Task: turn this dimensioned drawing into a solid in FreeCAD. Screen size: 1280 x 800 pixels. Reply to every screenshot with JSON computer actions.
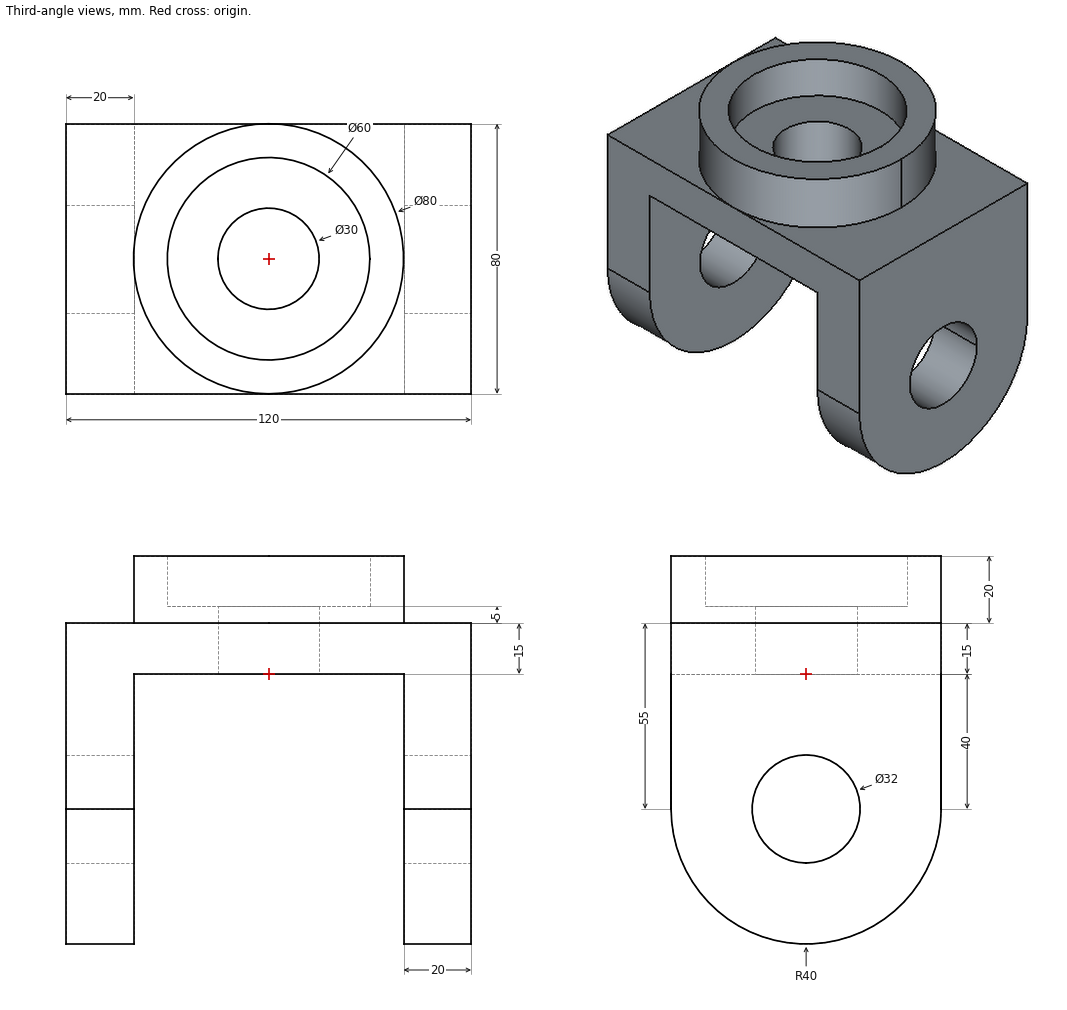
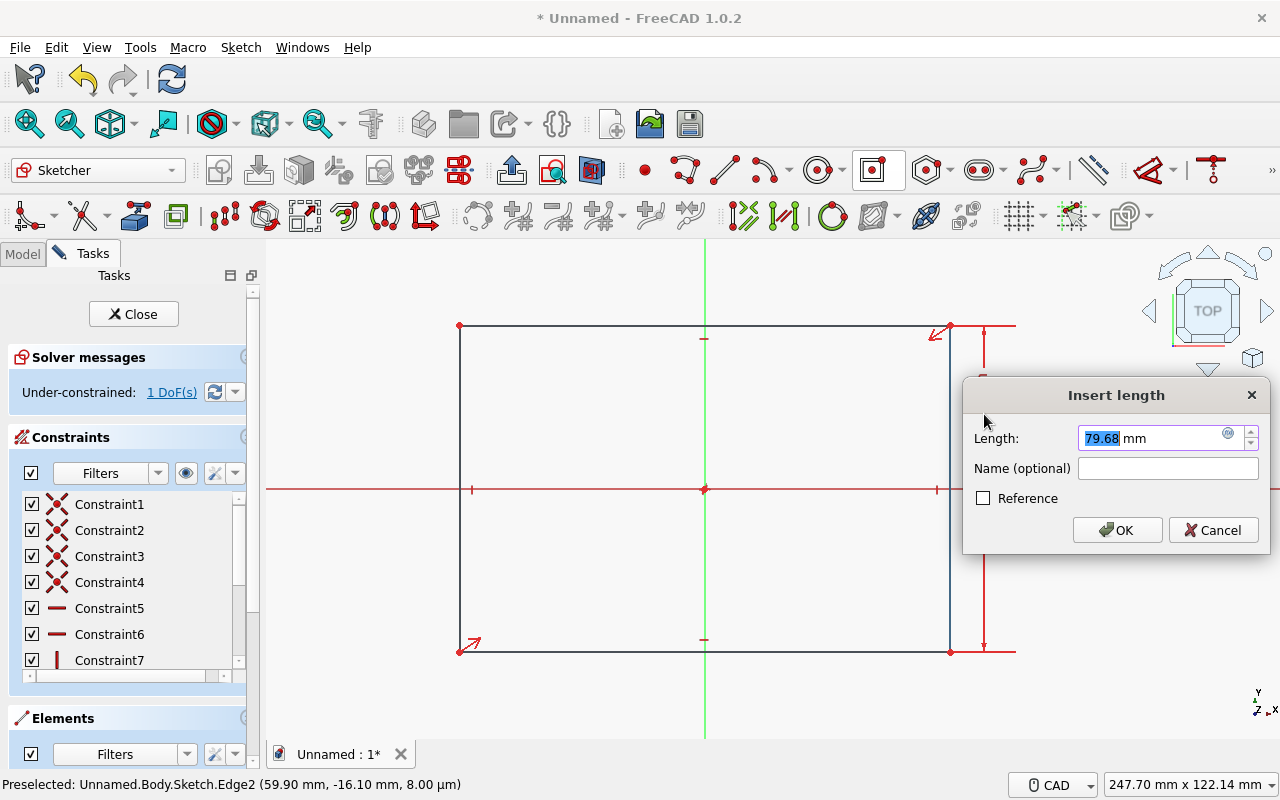
{"action": "type", "text": "80"}
{"action": "key", "text": "Return"}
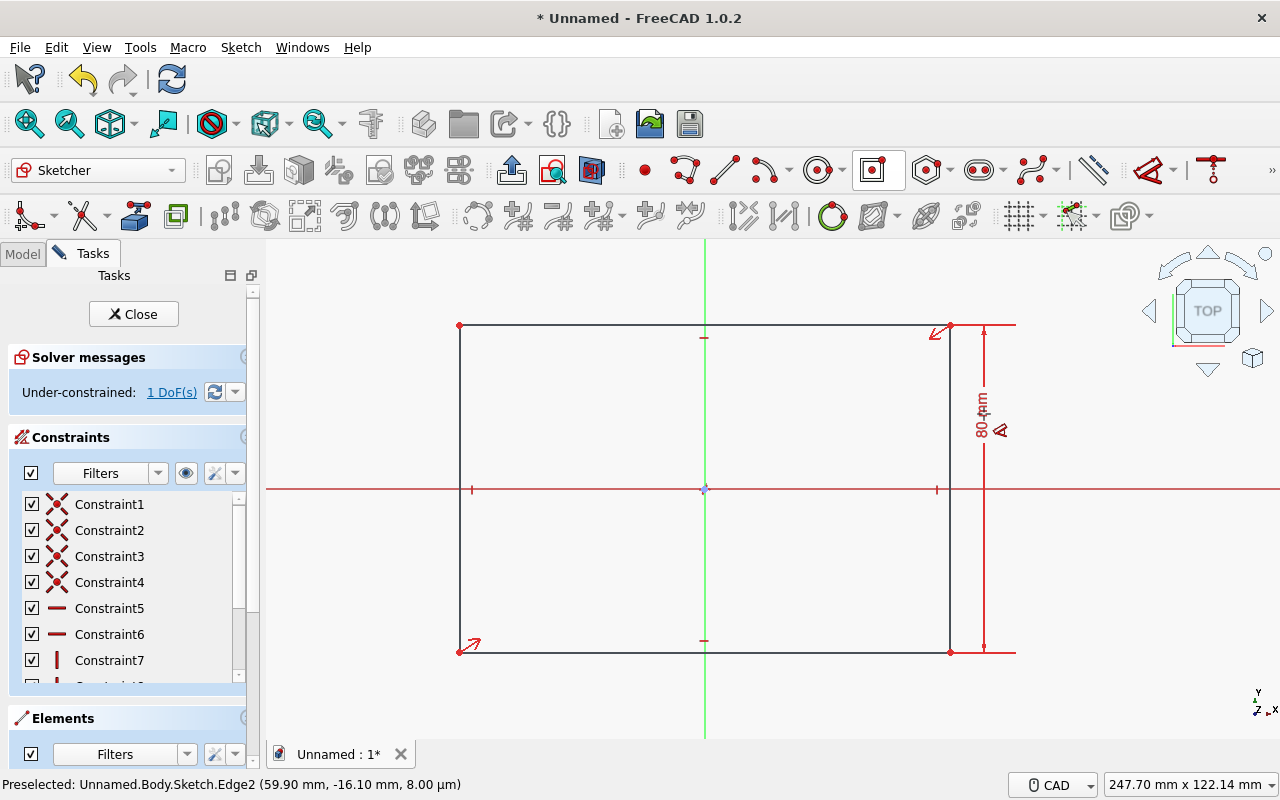
{"action": "left_click", "coordinate": [607, 653]}
{"action": "left_click", "coordinate": [592, 687]}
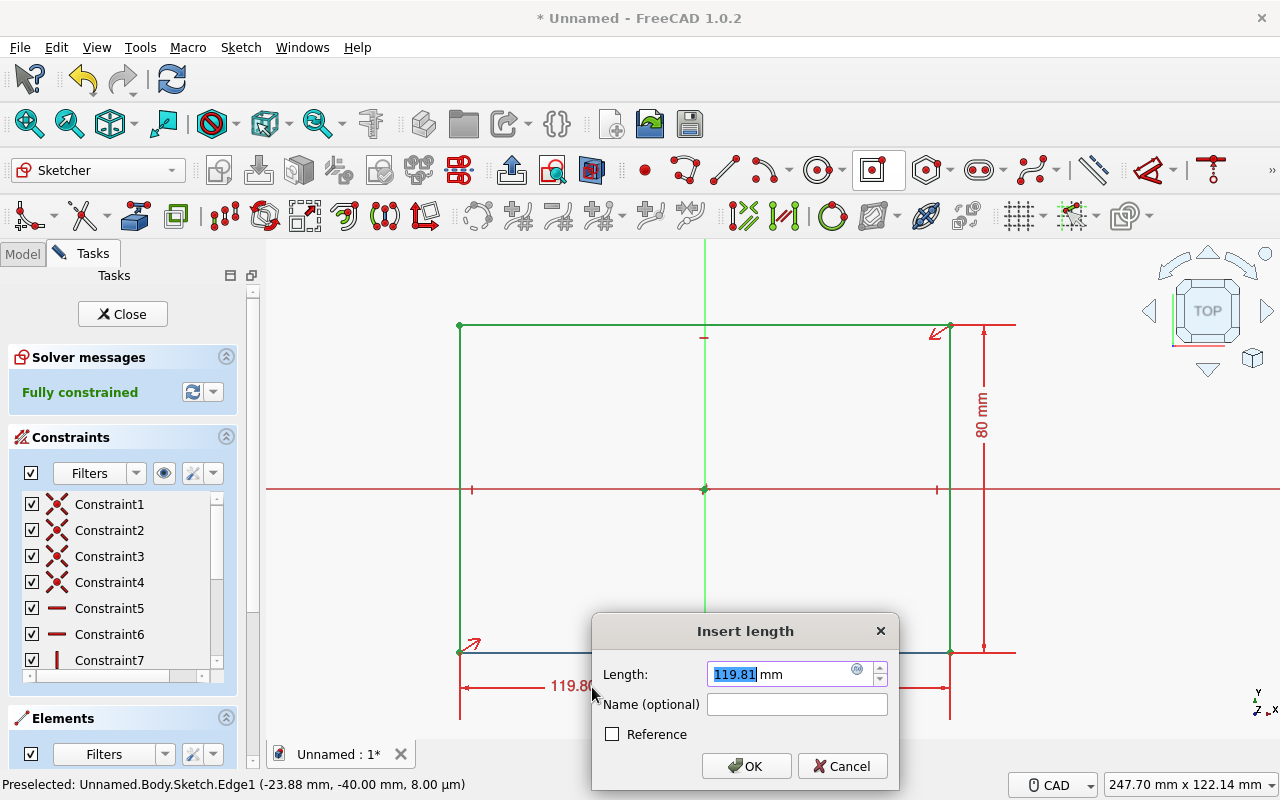
{"action": "type", "text": "120"}
{"action": "key", "text": "Return"}
{"action": "key", "text": "Escape"}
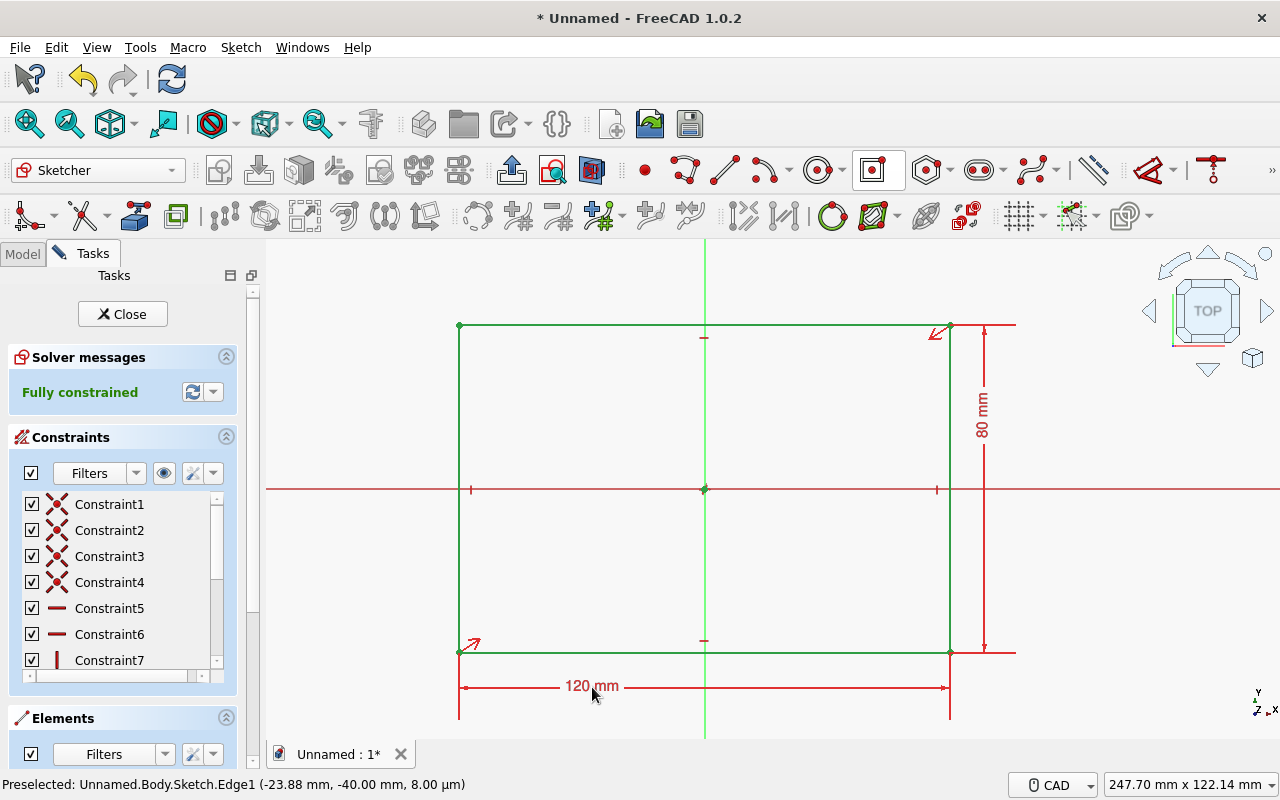
{"action": "left_click", "coordinate": [123, 314]}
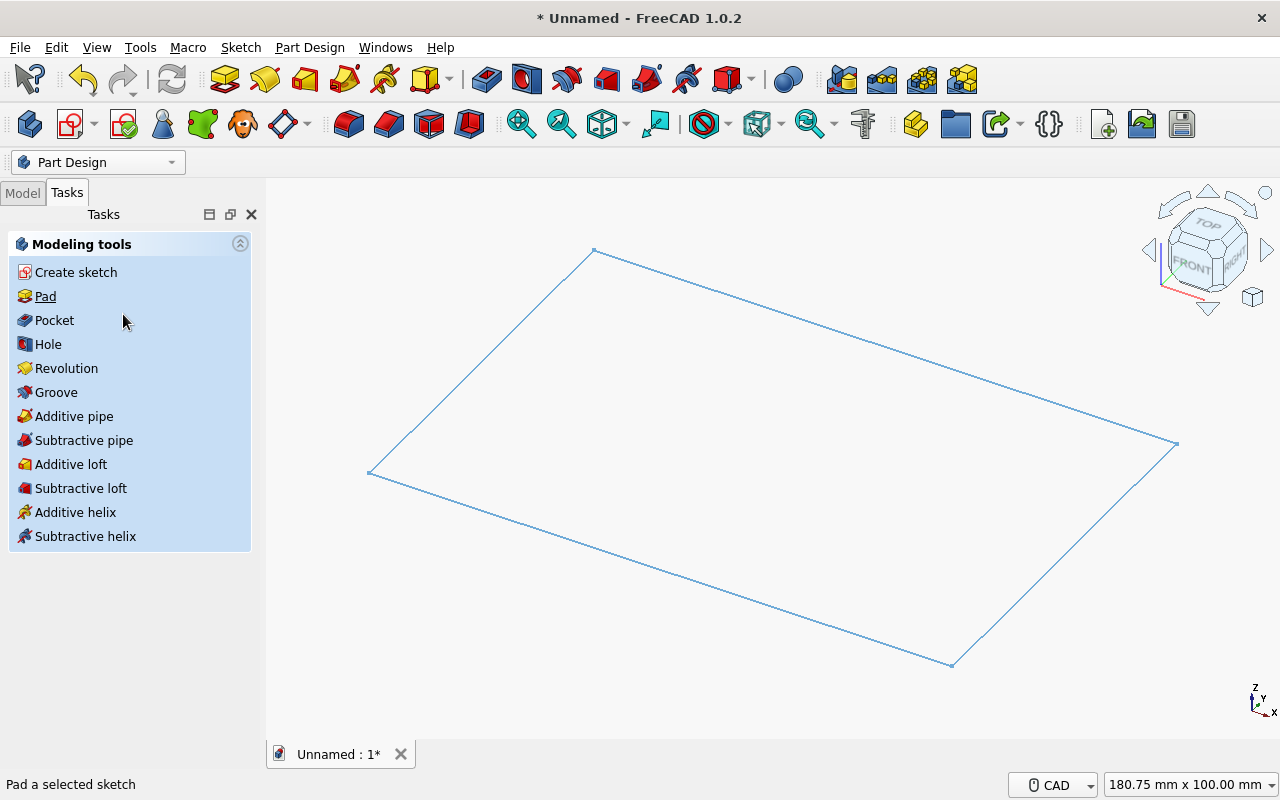
{"action": "left_click", "coordinate": [226, 80]}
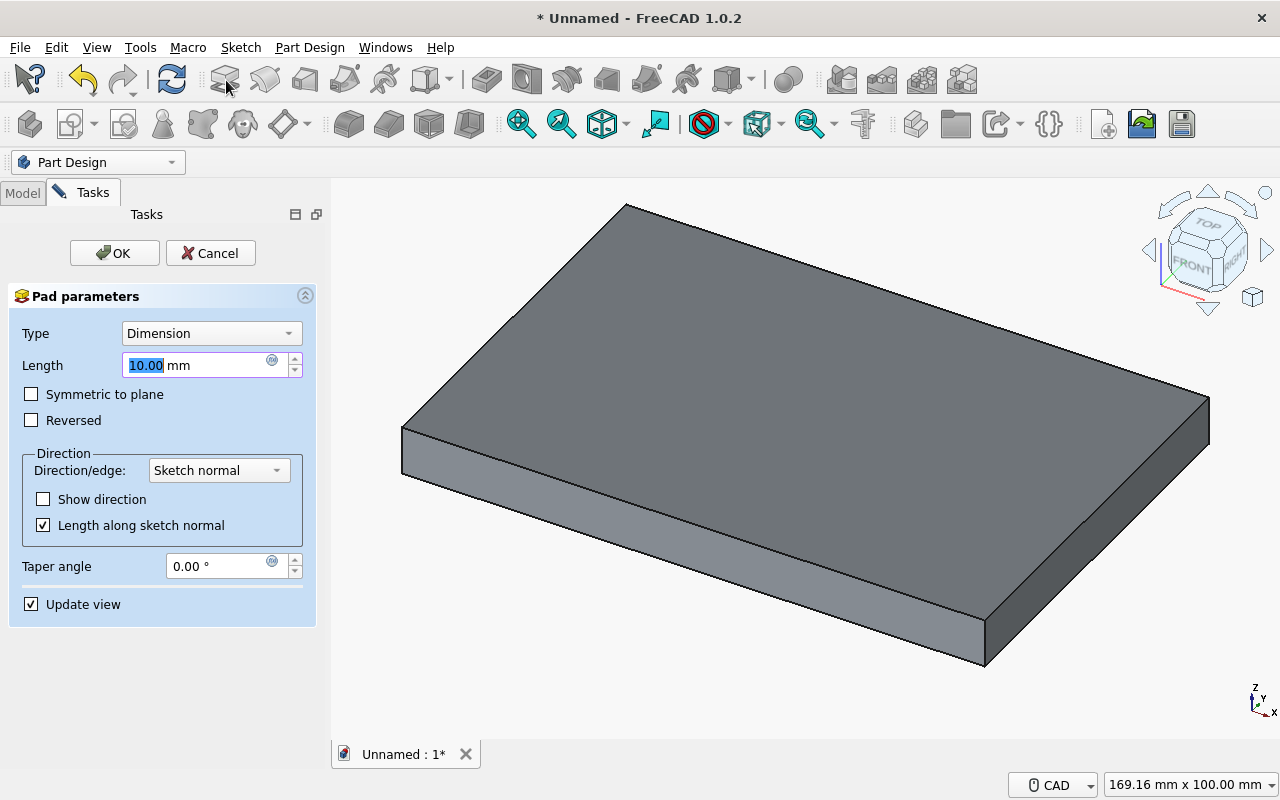
{"action": "type", "text": "15"}
{"action": "key", "text": "Tab"}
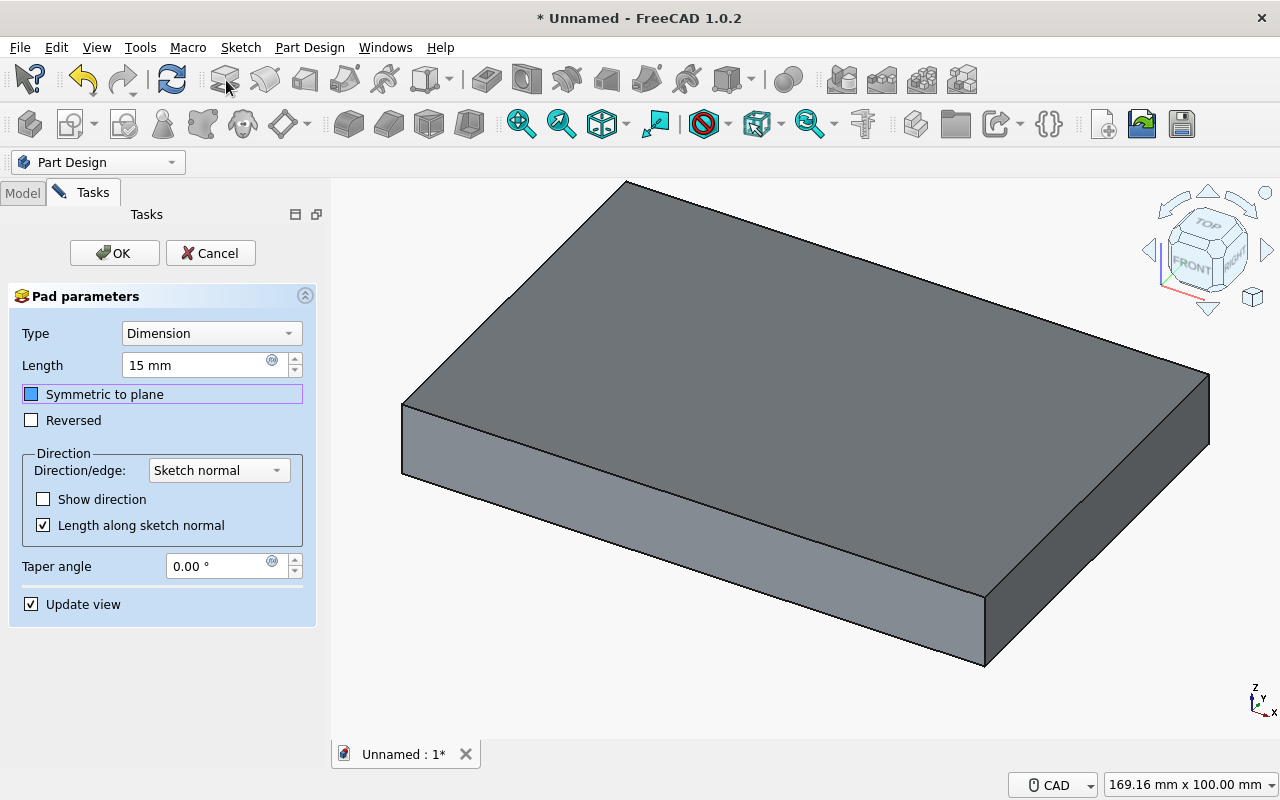
{"action": "left_click", "coordinate": [115, 253]}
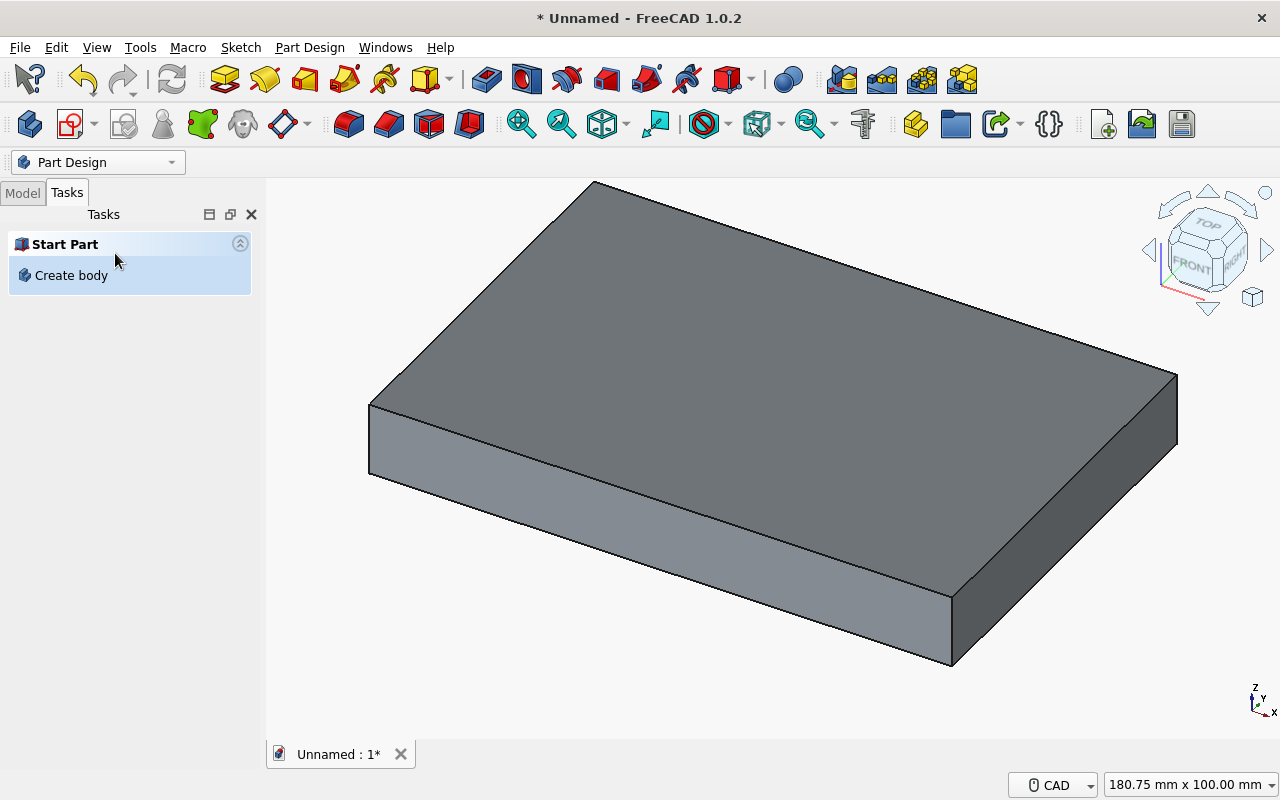
{"action": "left_click", "coordinate": [70, 124]}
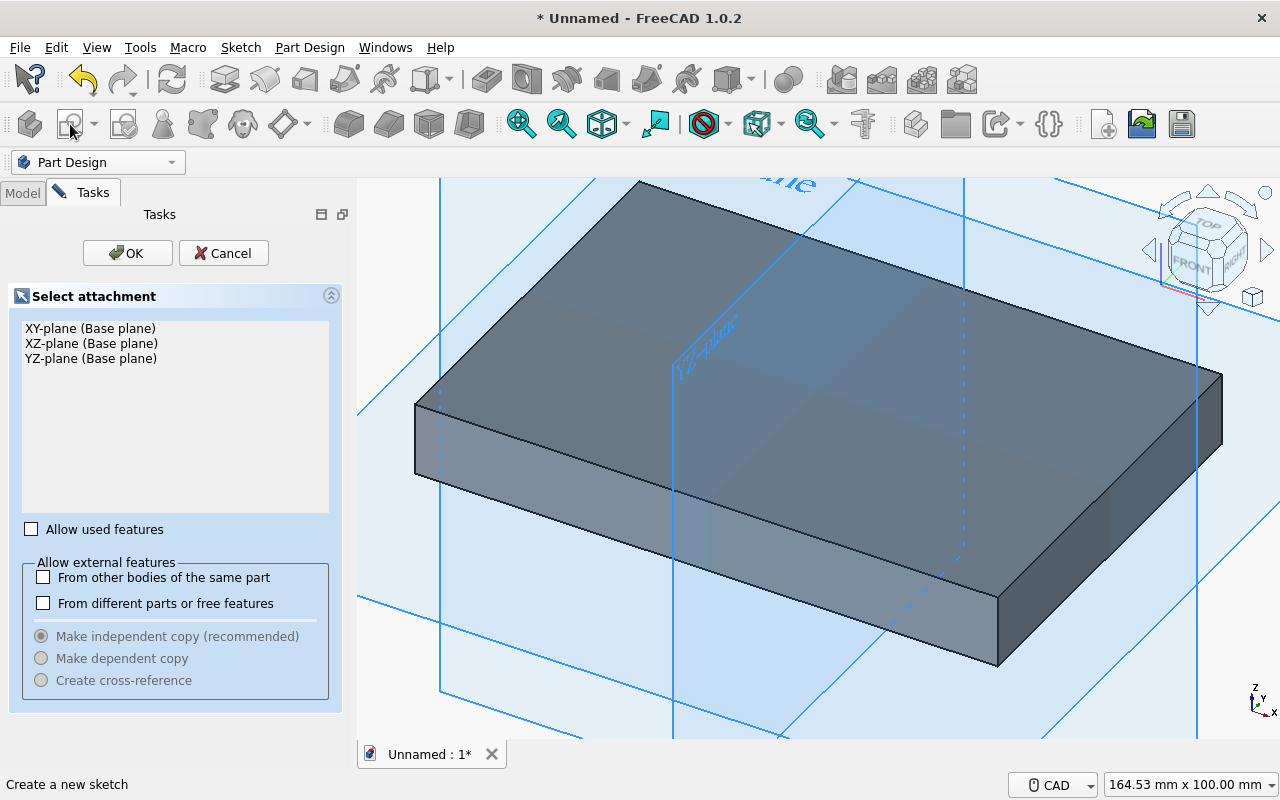
{"action": "left_click", "coordinate": [82, 328]}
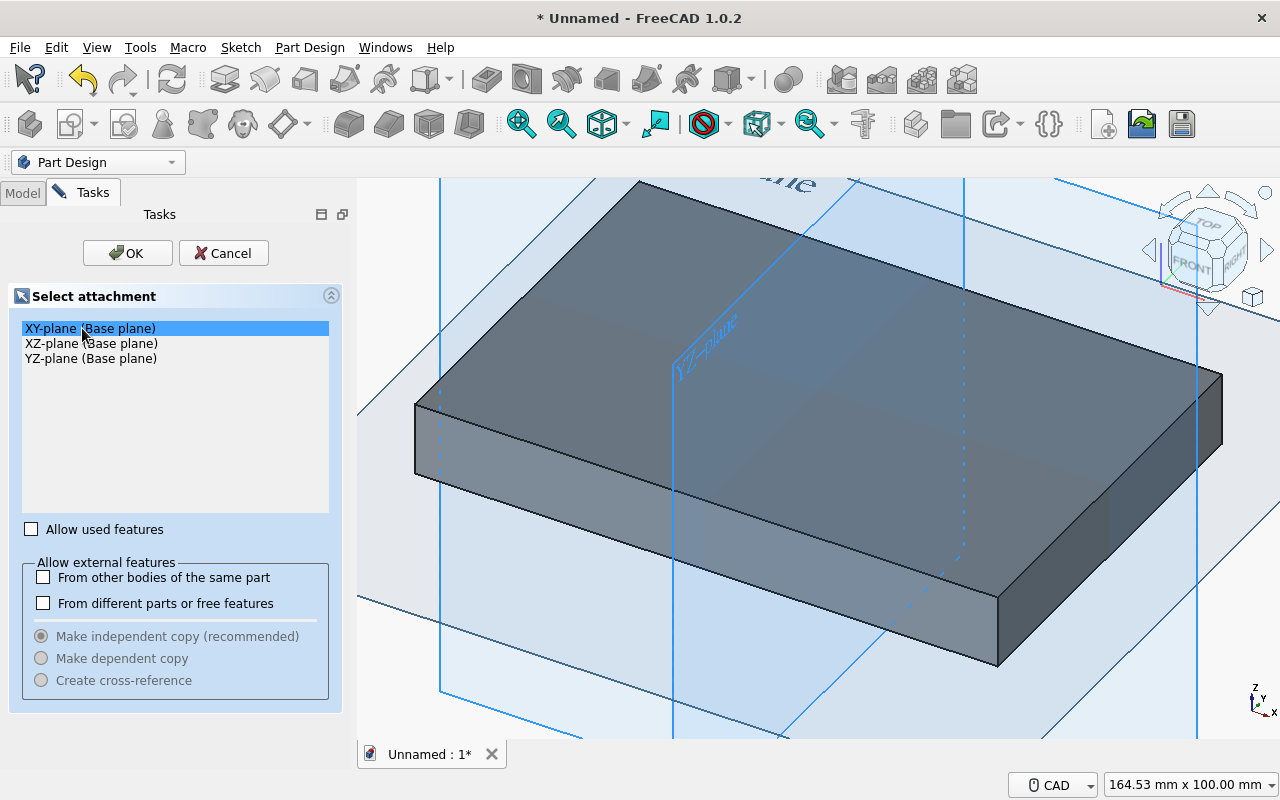
{"action": "left_click", "coordinate": [128, 253]}